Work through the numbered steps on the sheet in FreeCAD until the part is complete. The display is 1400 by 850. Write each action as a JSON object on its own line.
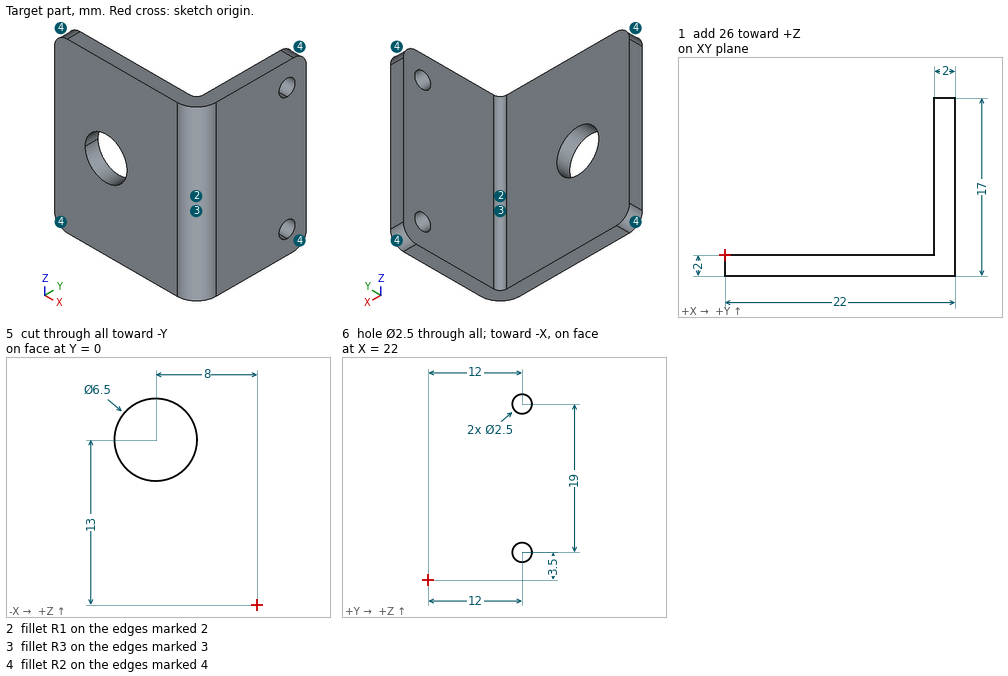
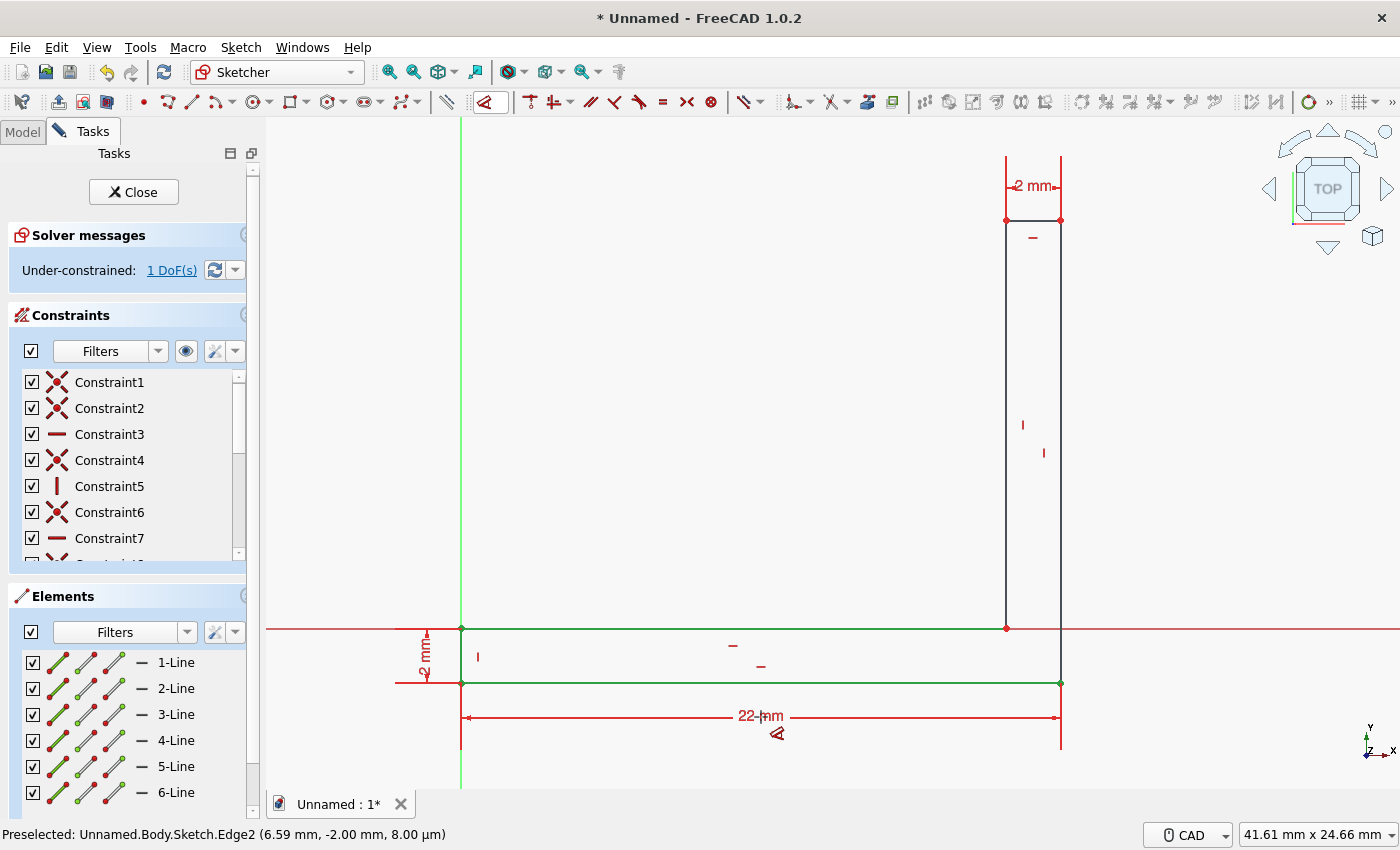
{"action": "left_click", "coordinate": [1061, 545]}
{"action": "left_click", "coordinate": [1095, 452]}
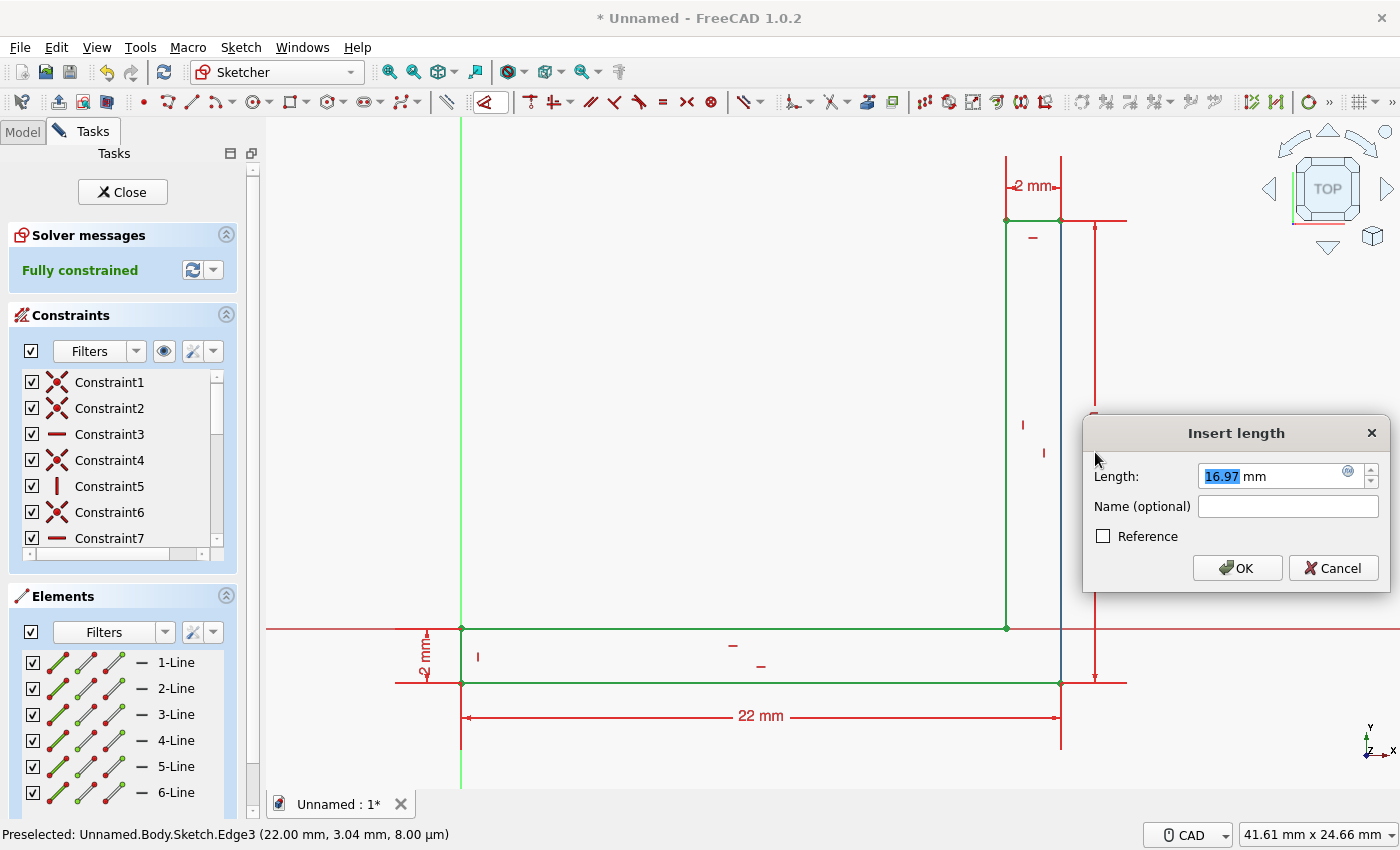
{"action": "type", "text": "17"}
{"action": "key", "text": "Return"}
{"action": "key", "text": "Escape"}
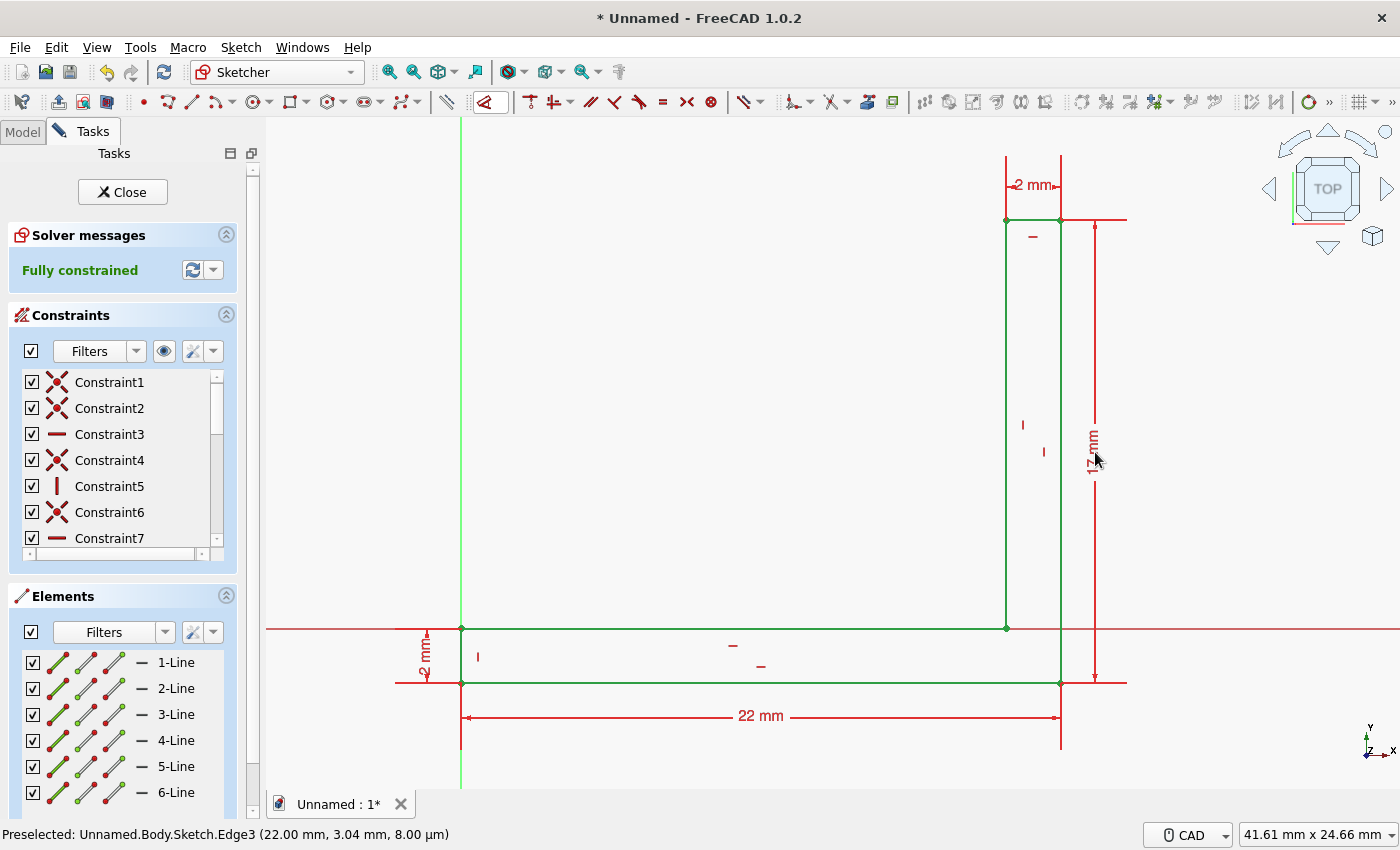
{"action": "left_click", "coordinate": [123, 192]}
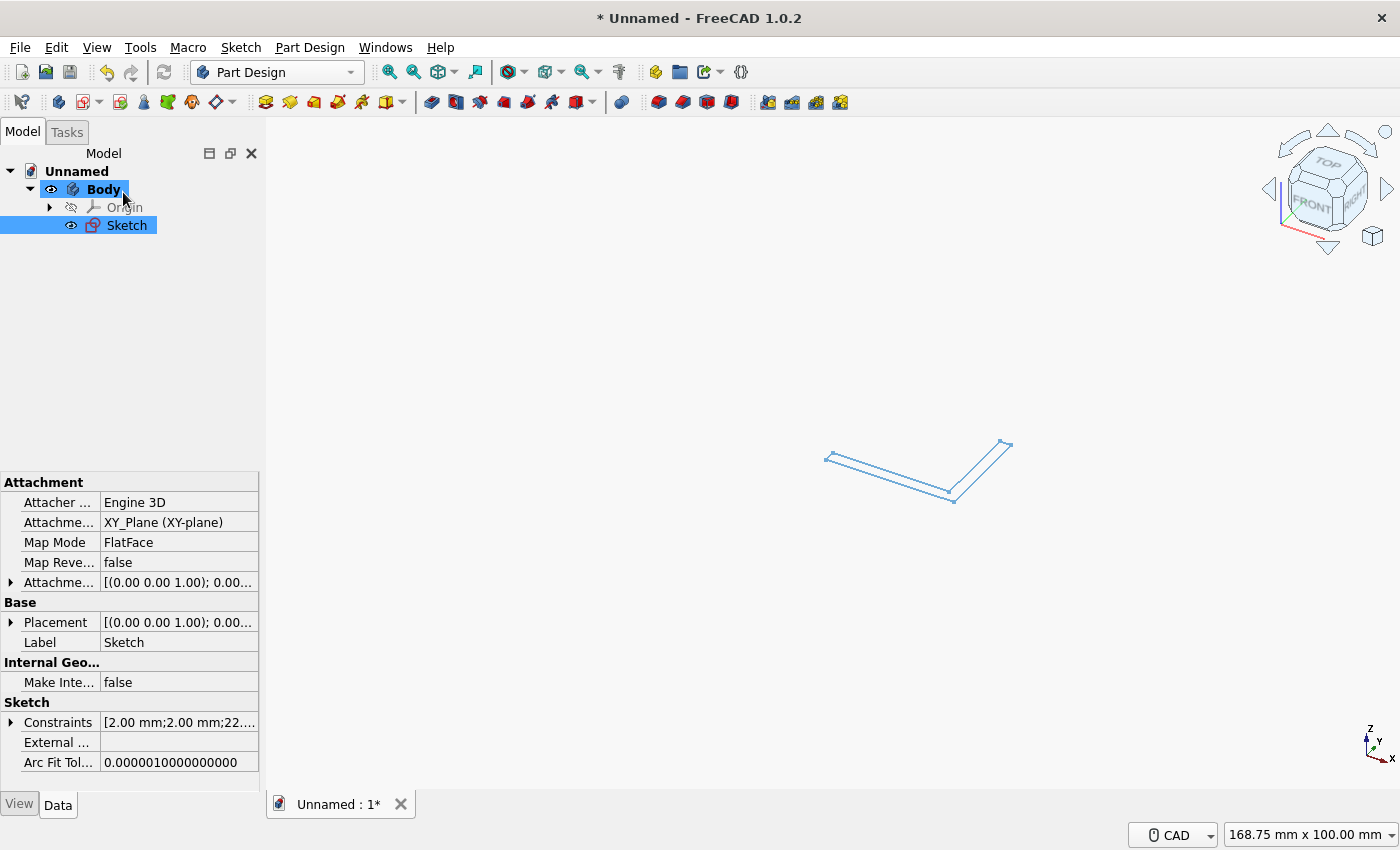
{"action": "left_click", "coordinate": [266, 102]}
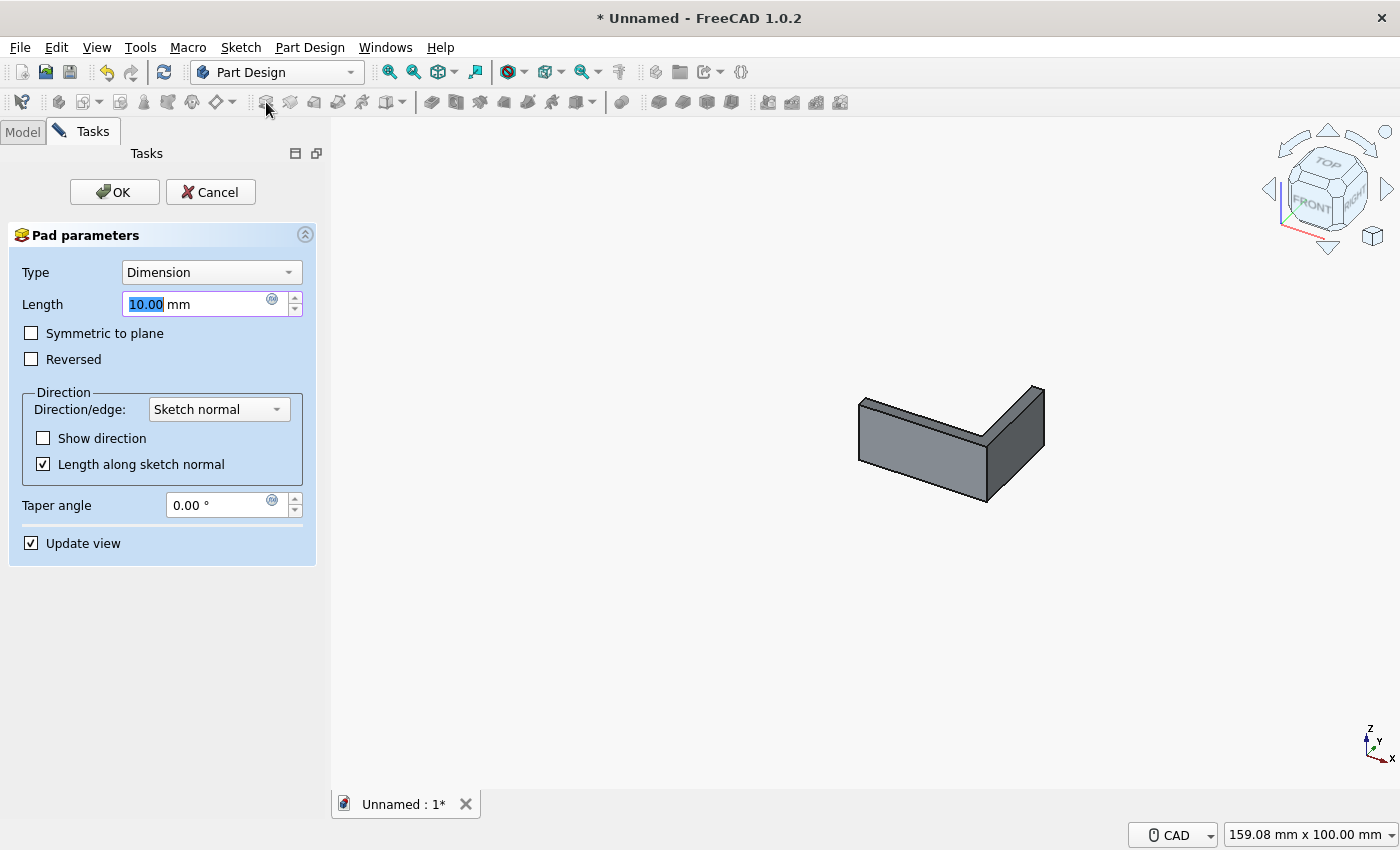
{"action": "type", "text": "26"}
{"action": "key", "text": "Tab"}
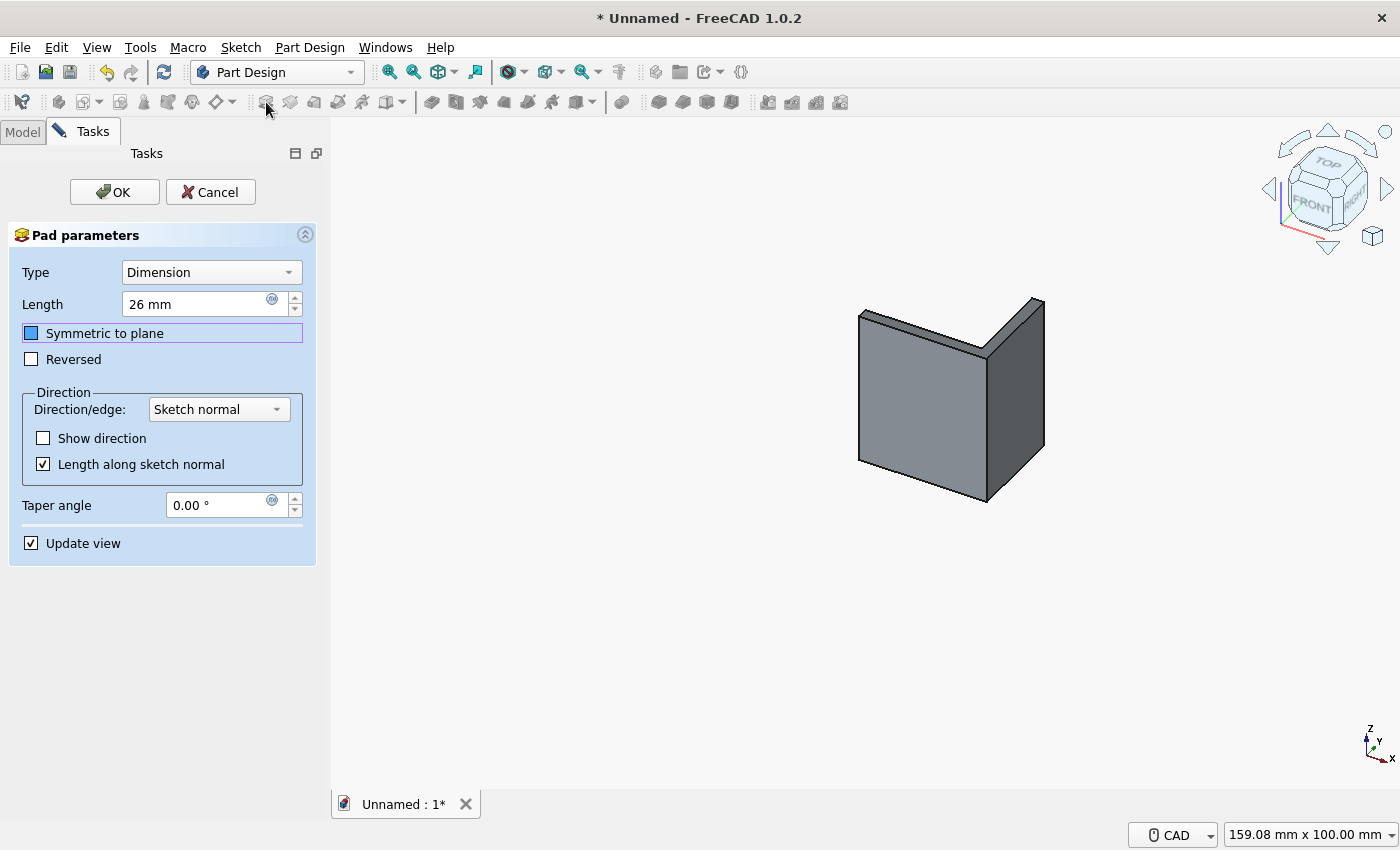
{"action": "left_click", "coordinate": [115, 192]}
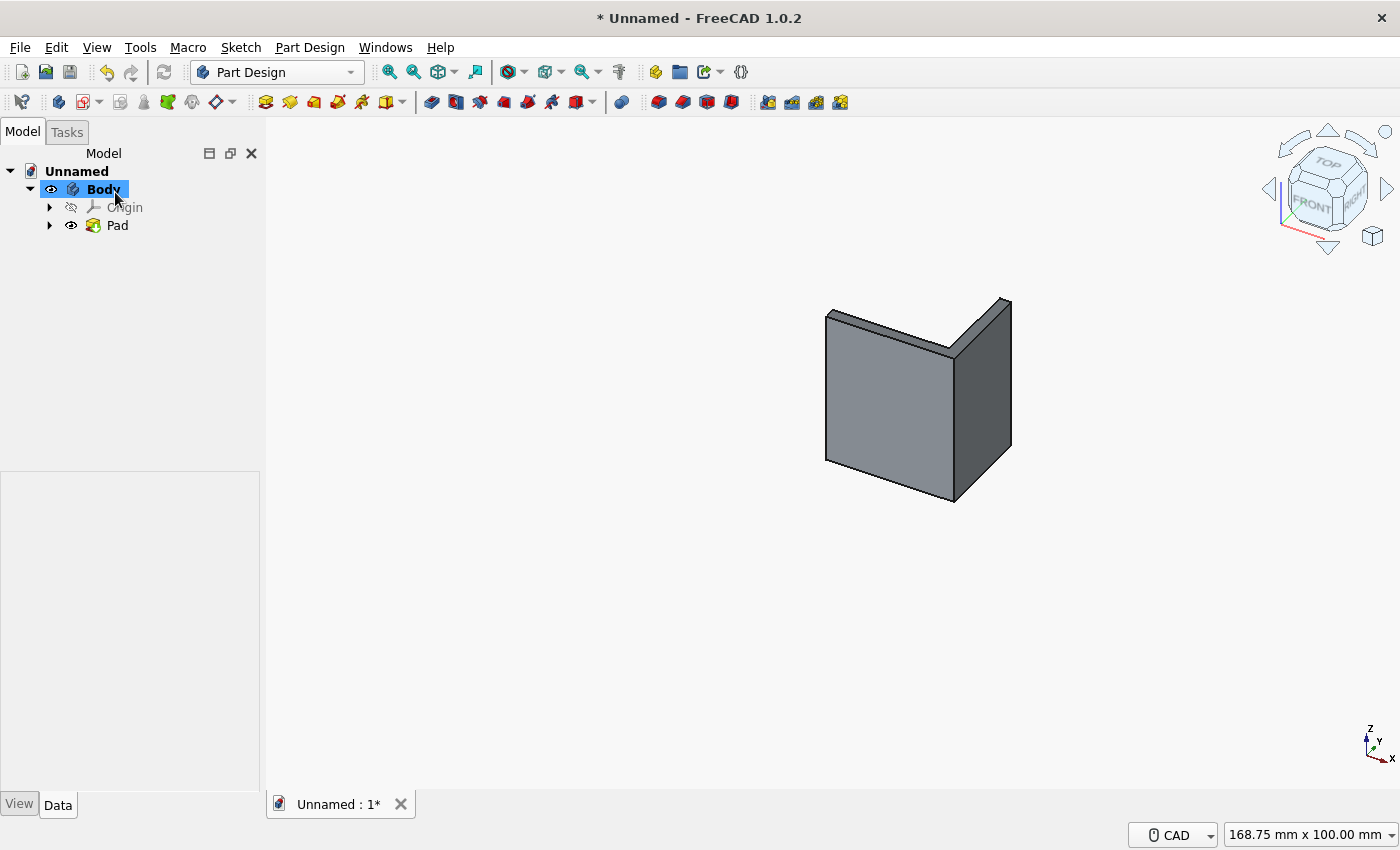
{"action": "key", "text": "v f"}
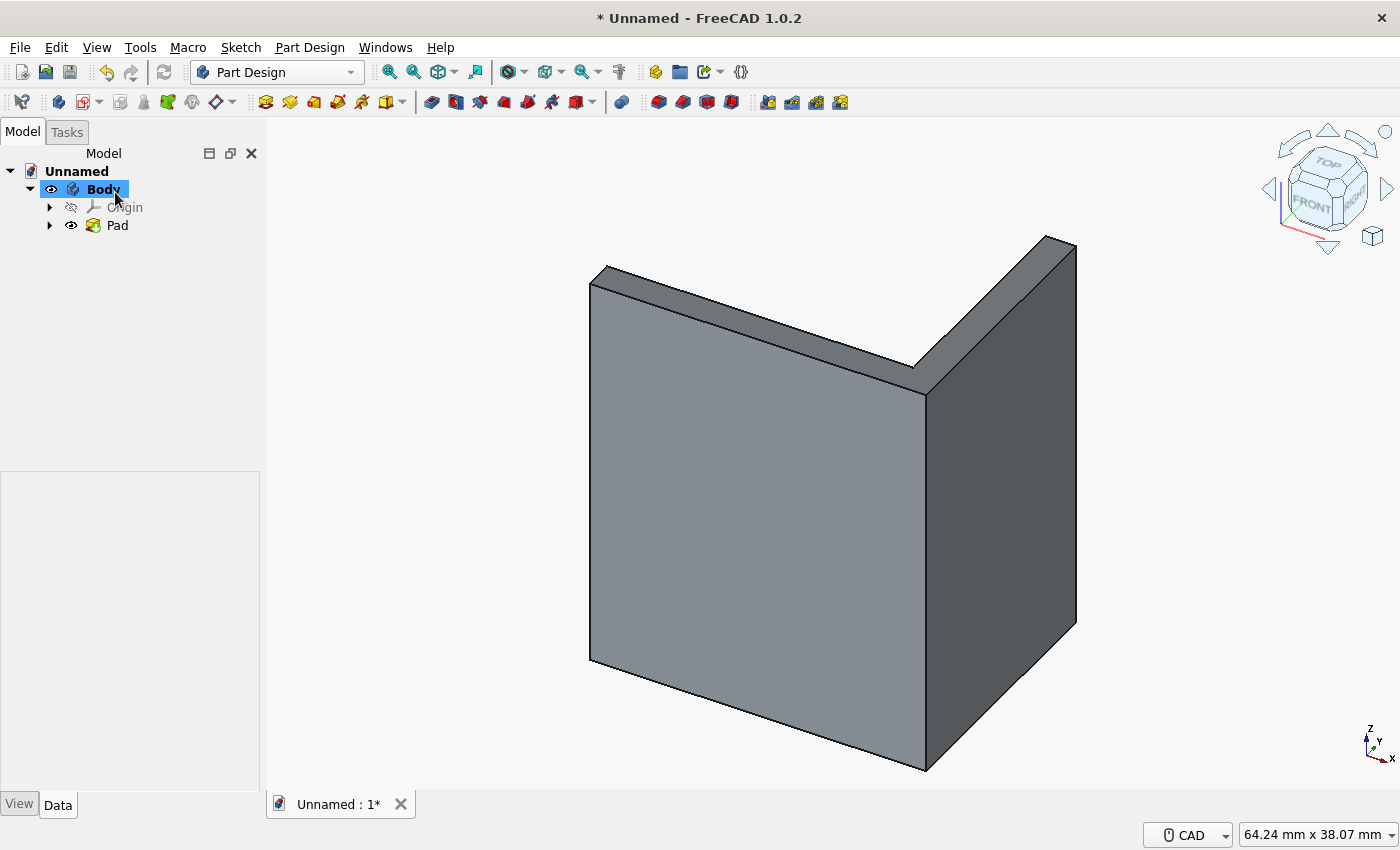
{"action": "key", "text": "0"}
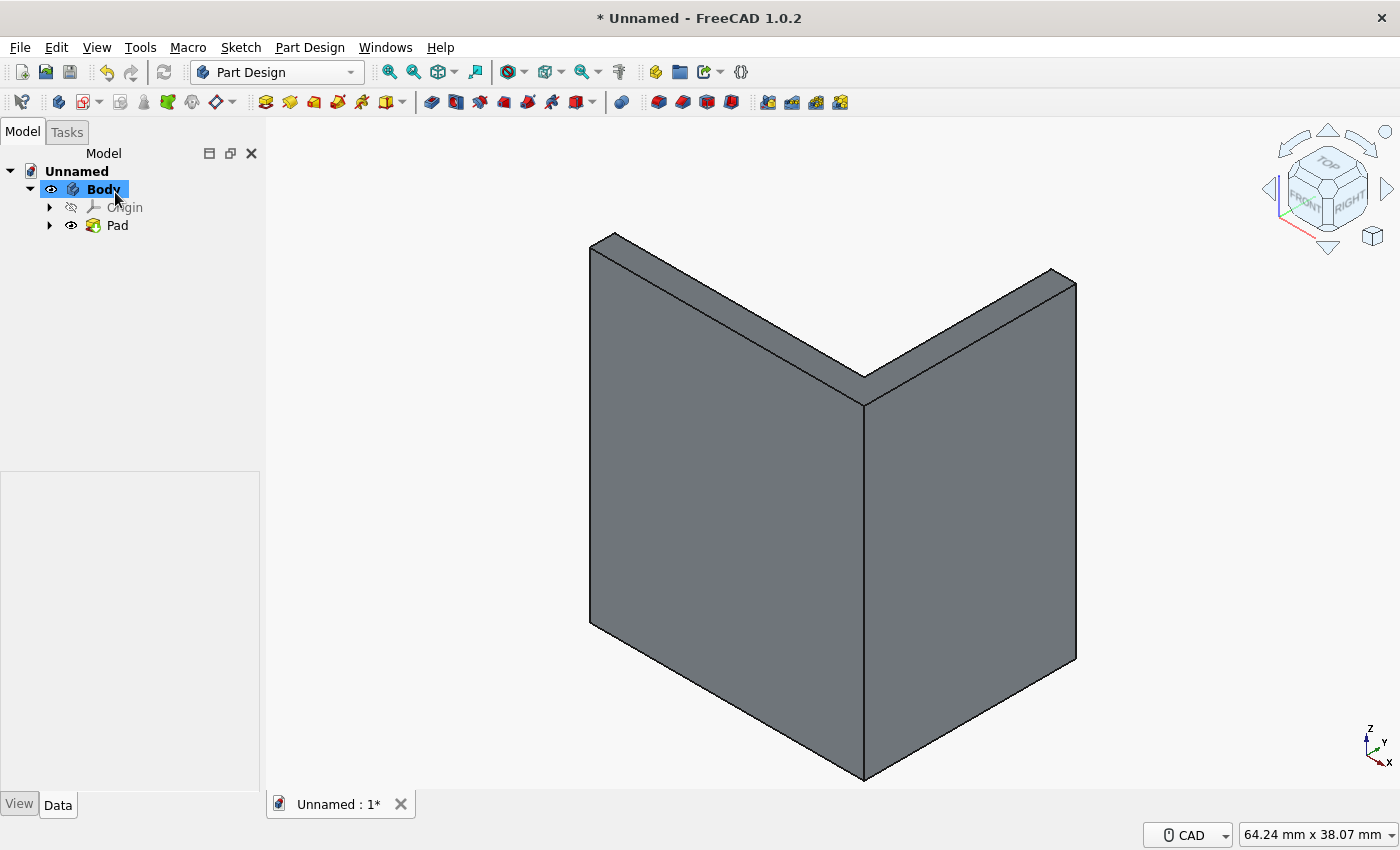
{"action": "key", "text": "2"}